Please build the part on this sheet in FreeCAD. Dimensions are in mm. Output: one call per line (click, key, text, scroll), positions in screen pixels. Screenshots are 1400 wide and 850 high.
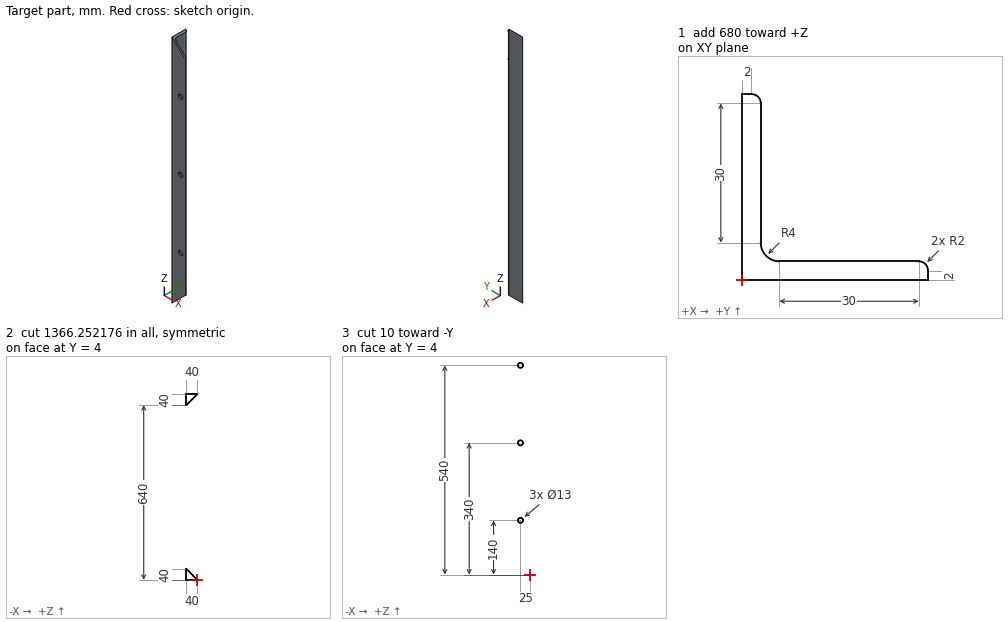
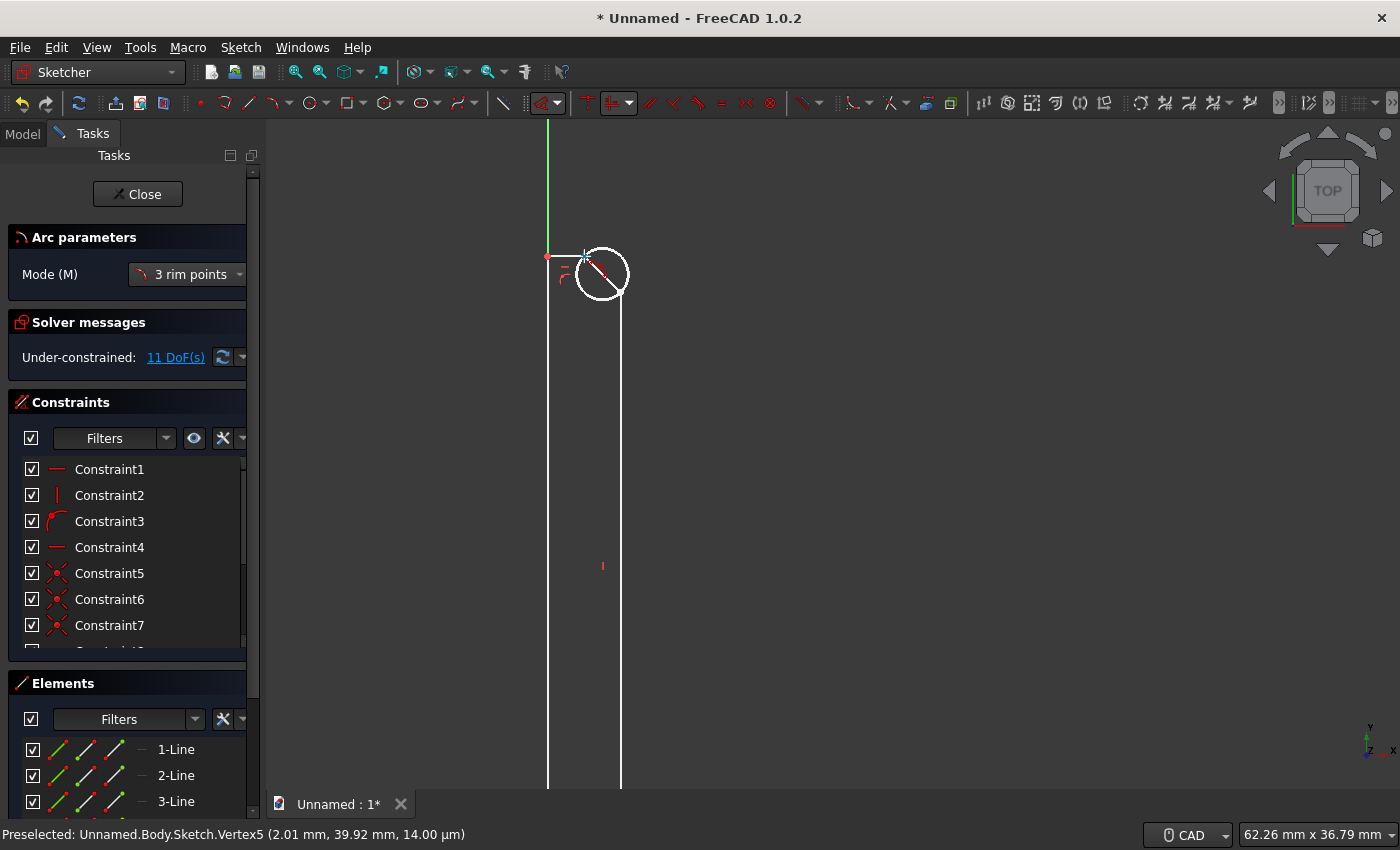
scroll(610, 265, up, 2)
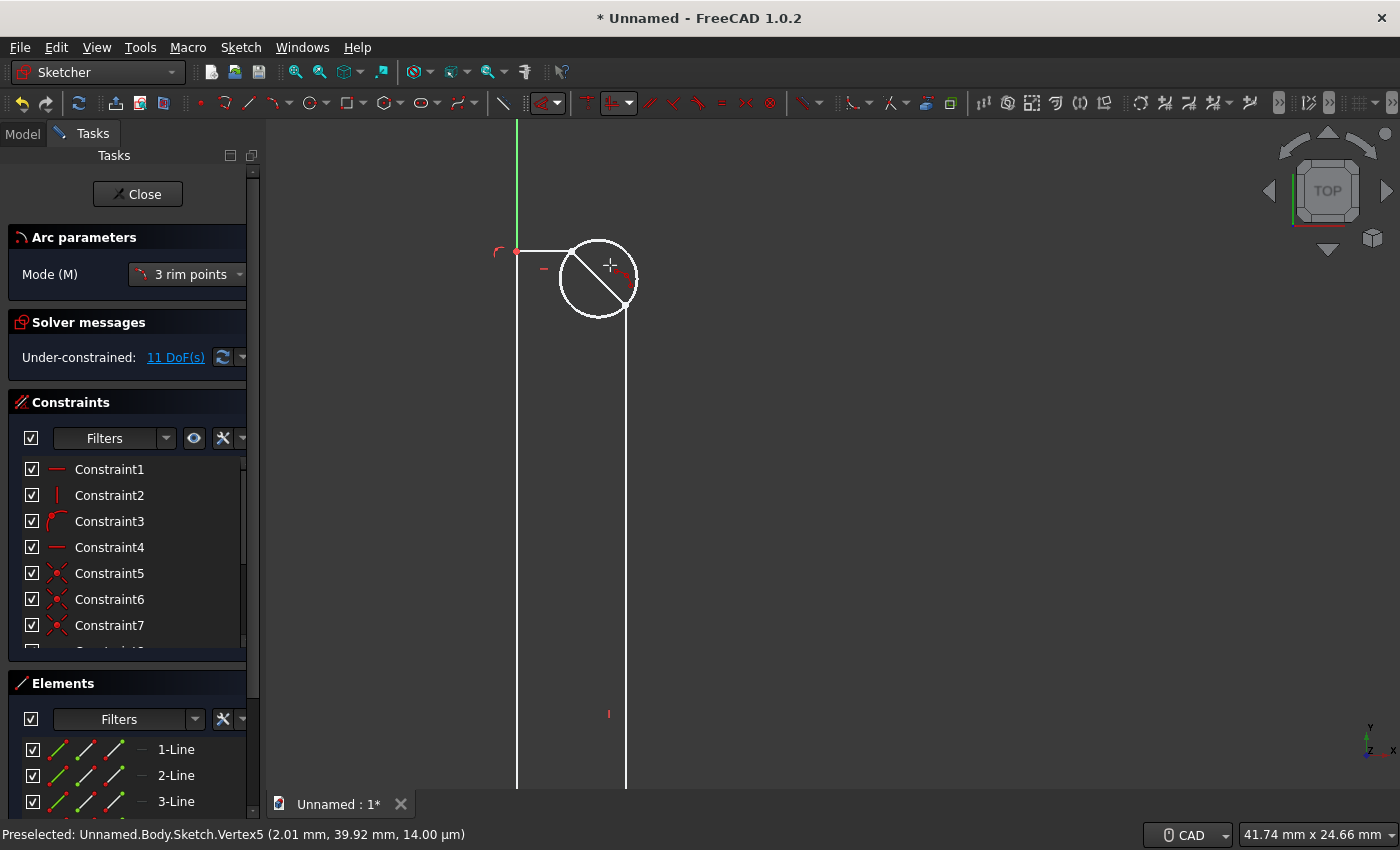
click(609, 265)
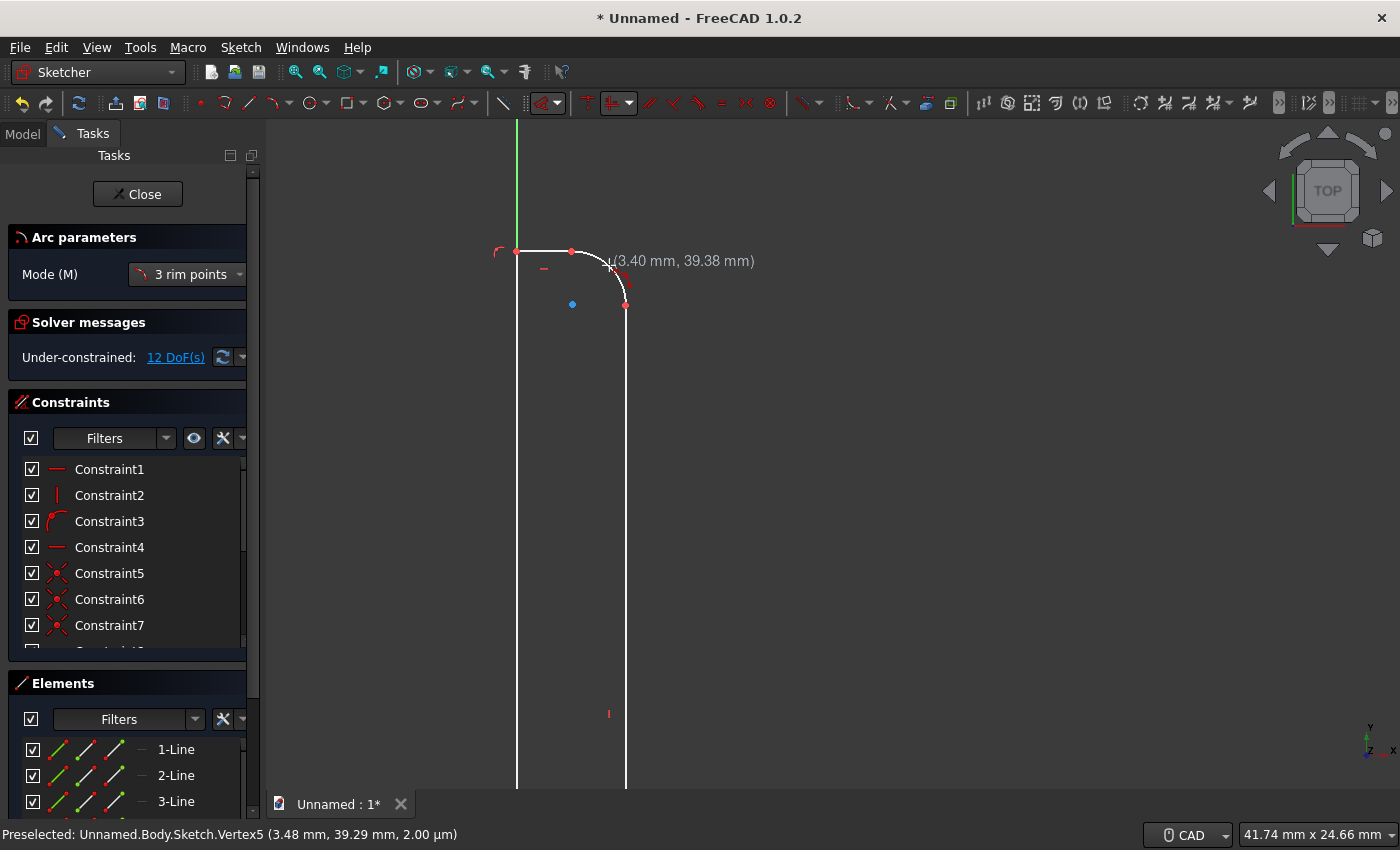
scroll(592, 257, down, 5)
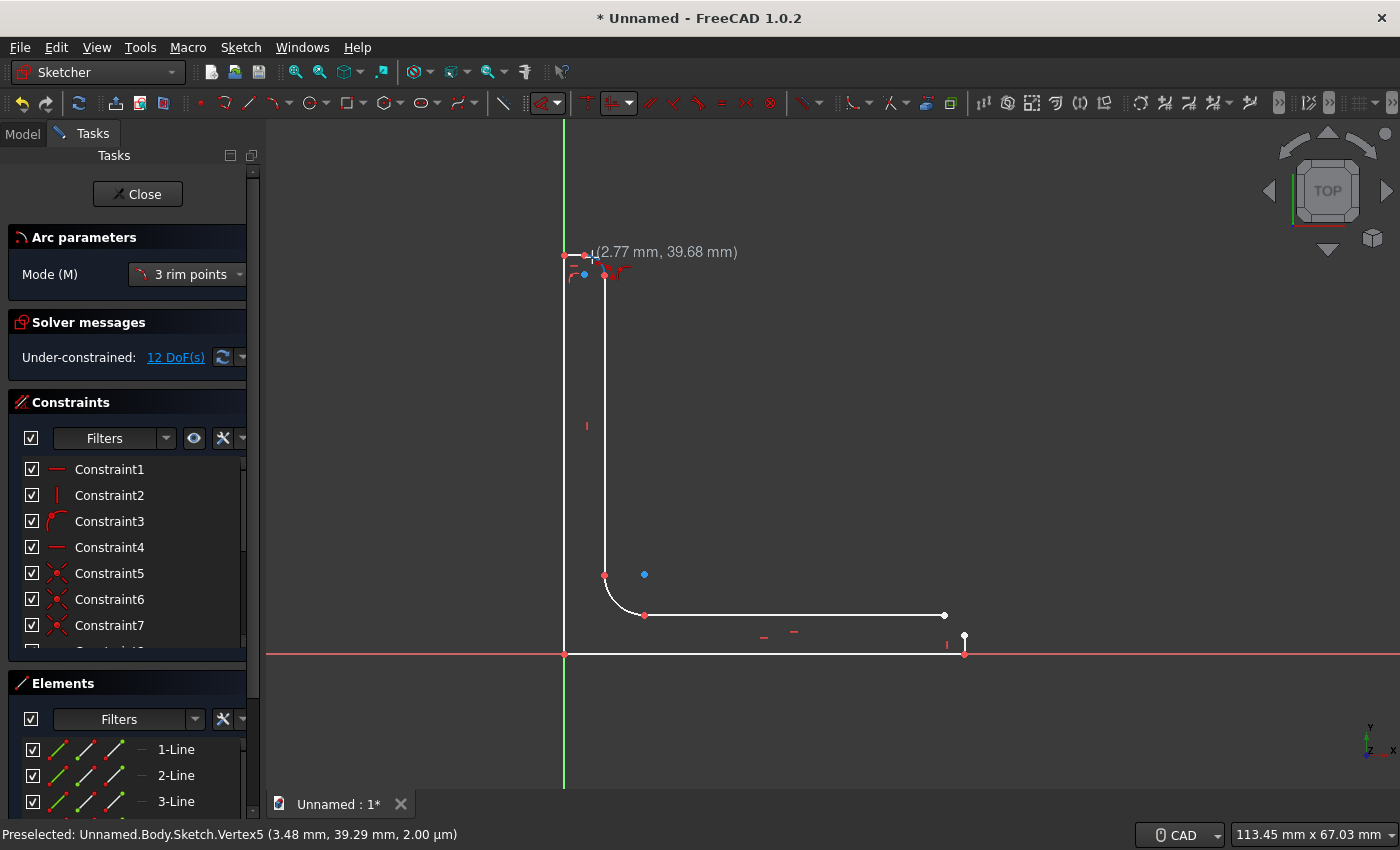
scroll(964, 634, up, 3)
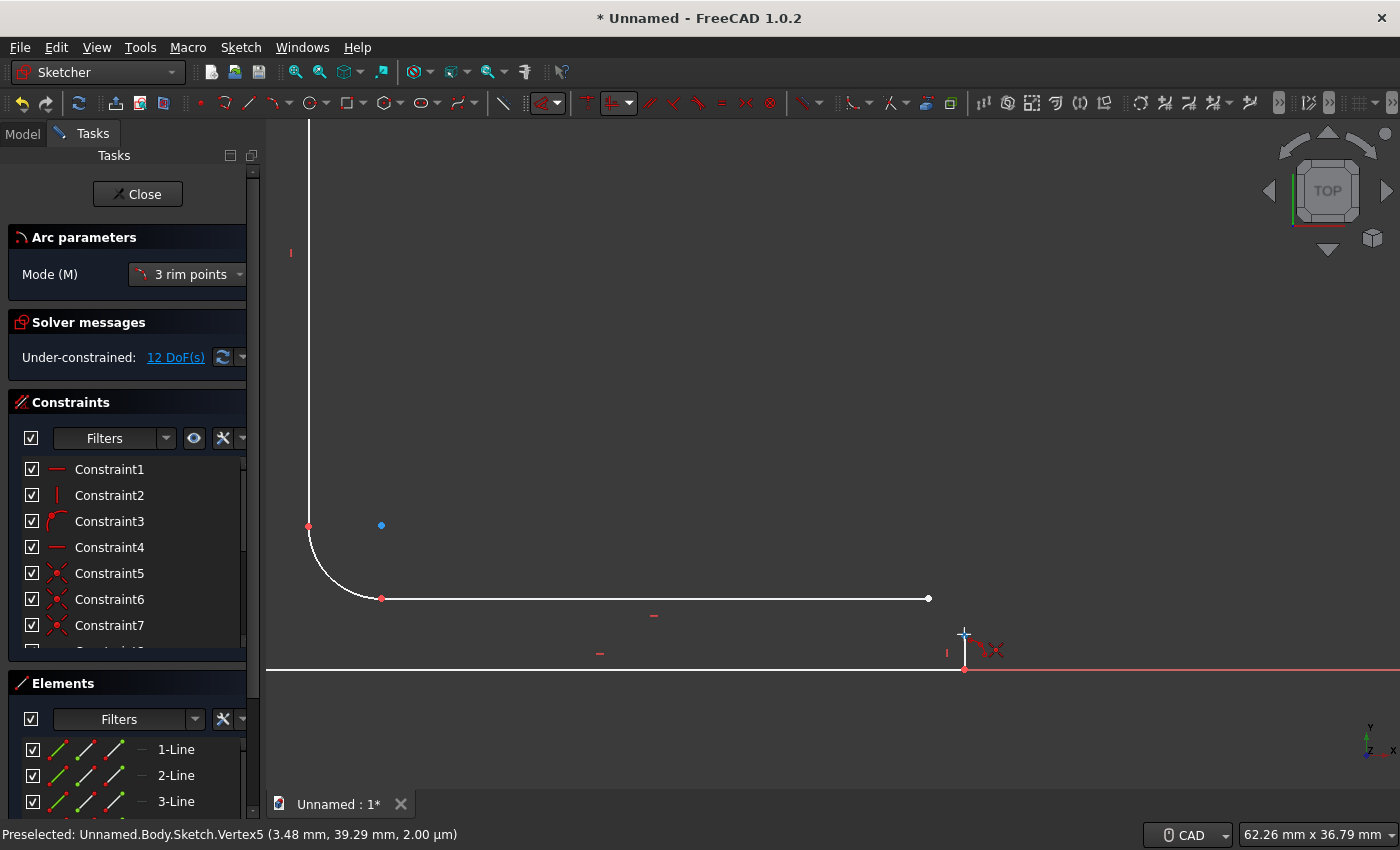
click(965, 635)
click(928, 599)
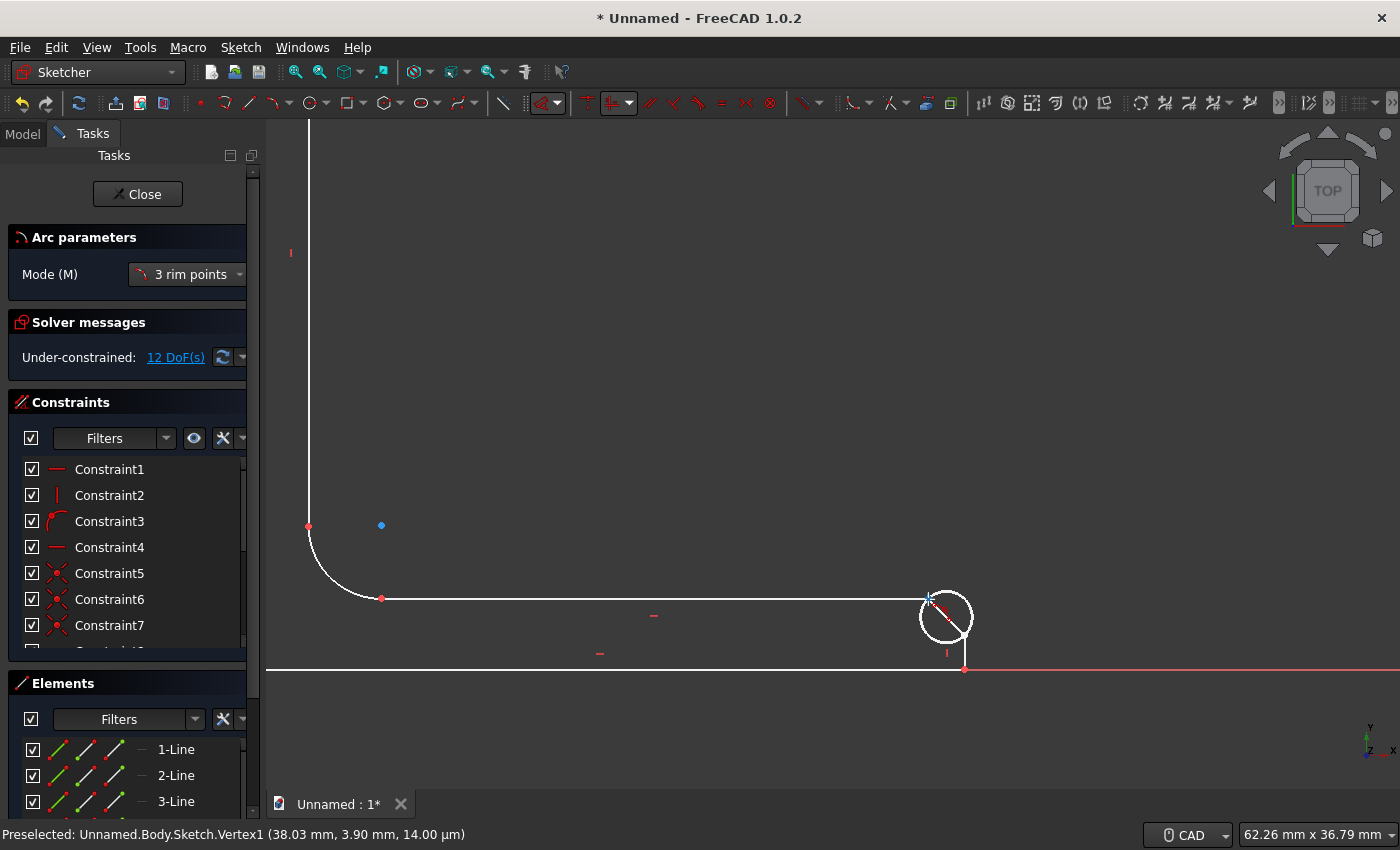
scroll(953, 608, up, 2)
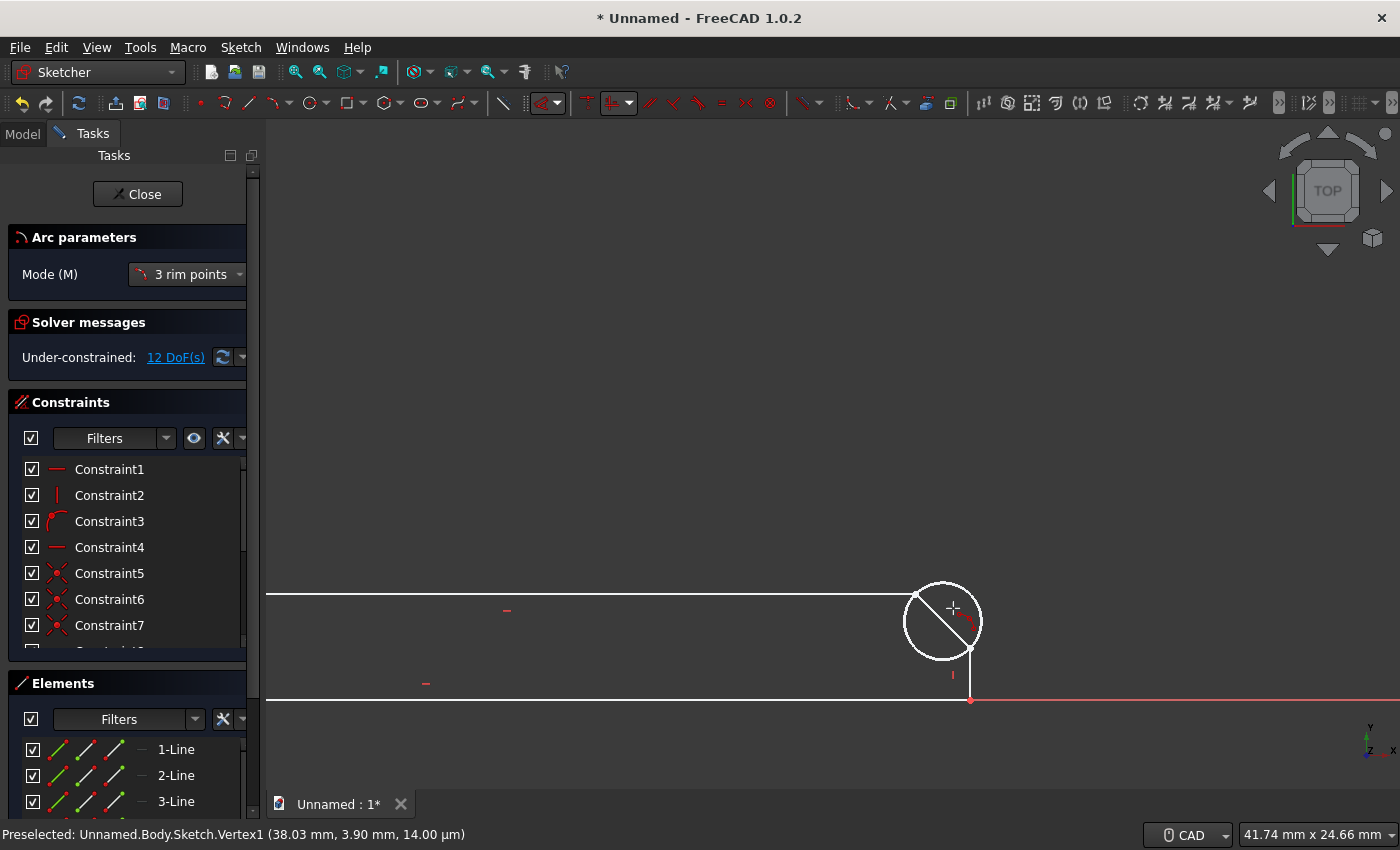
click(953, 607)
key(Escape)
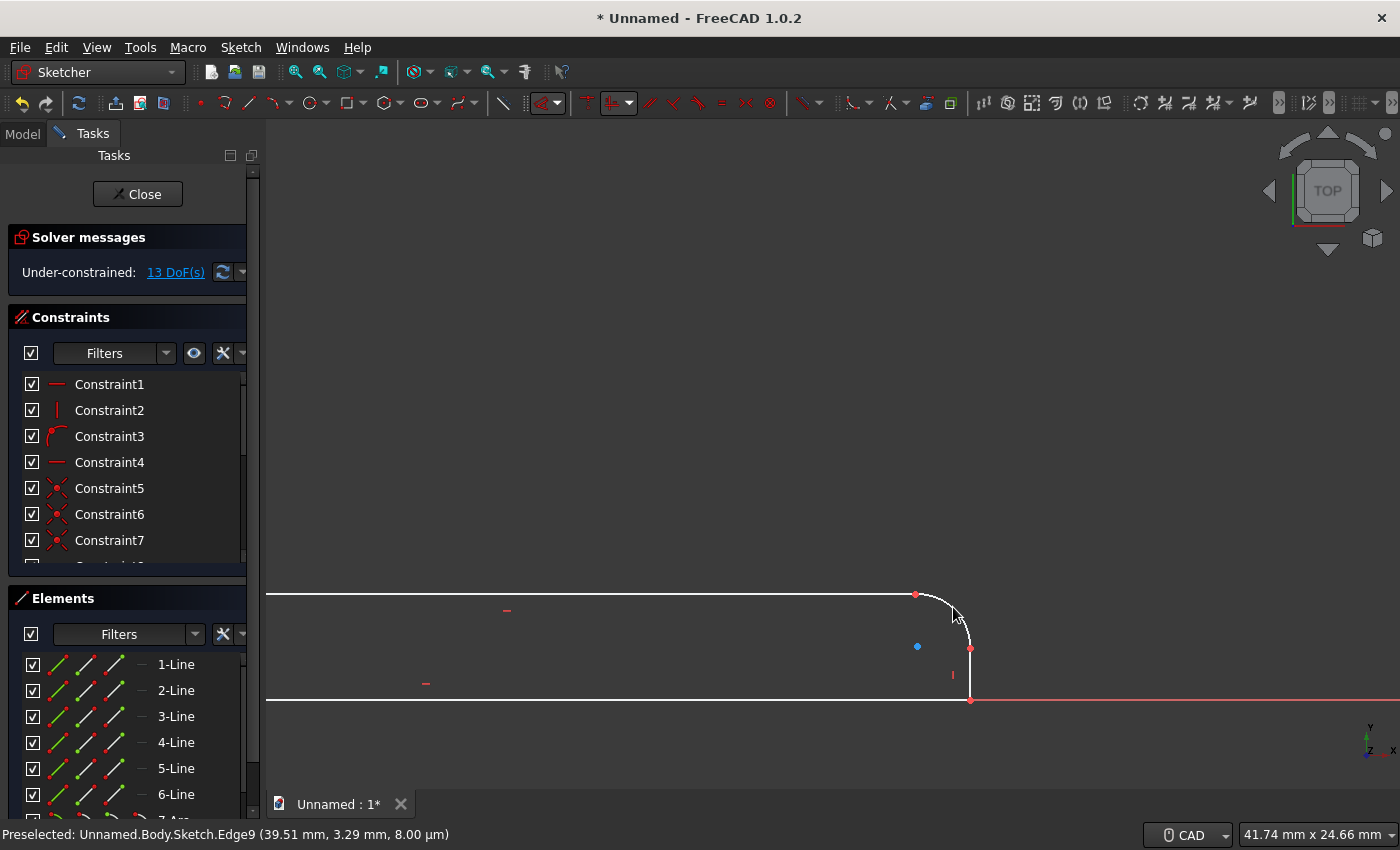
click(671, 594)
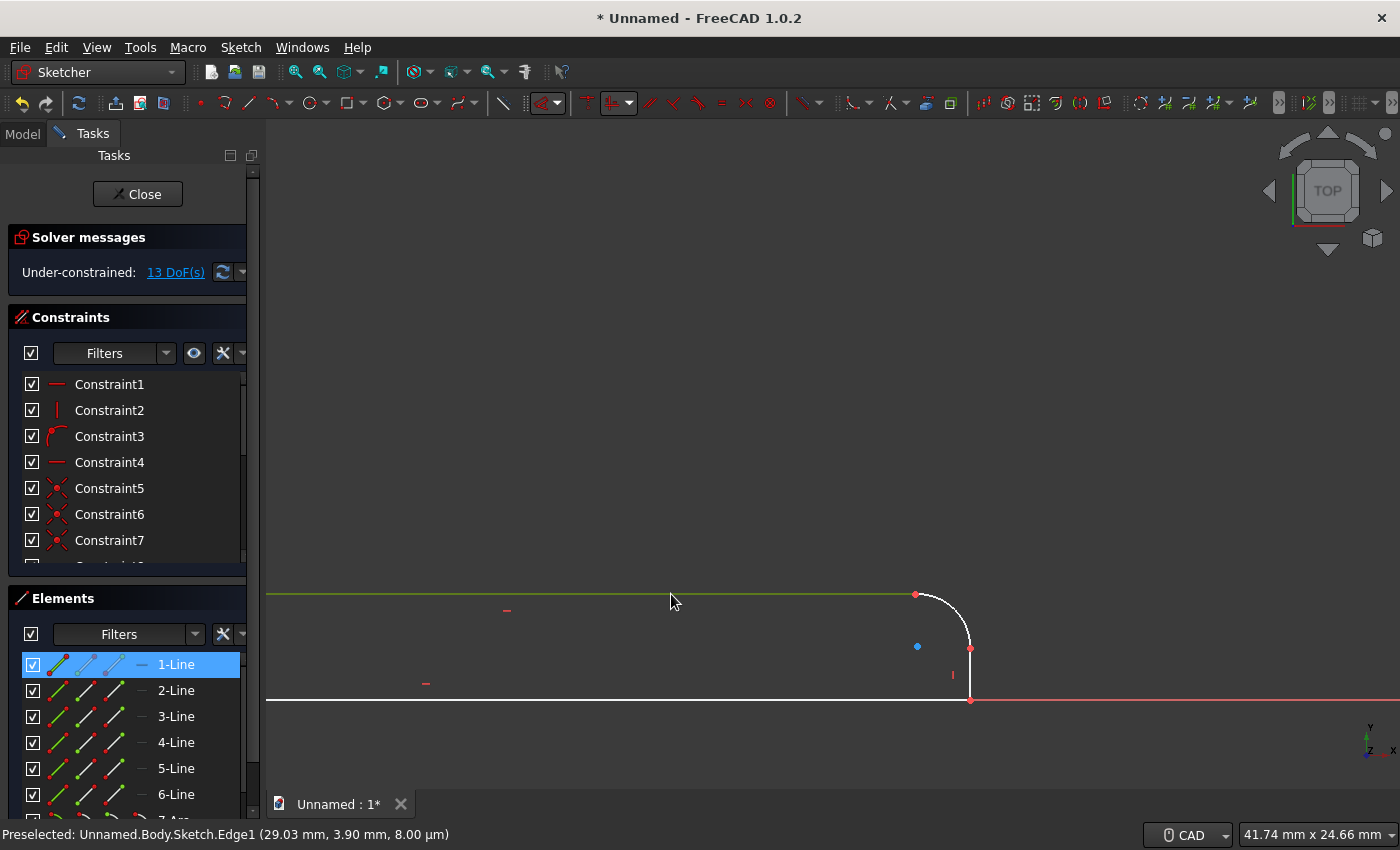
scroll(962, 627, down, 5)